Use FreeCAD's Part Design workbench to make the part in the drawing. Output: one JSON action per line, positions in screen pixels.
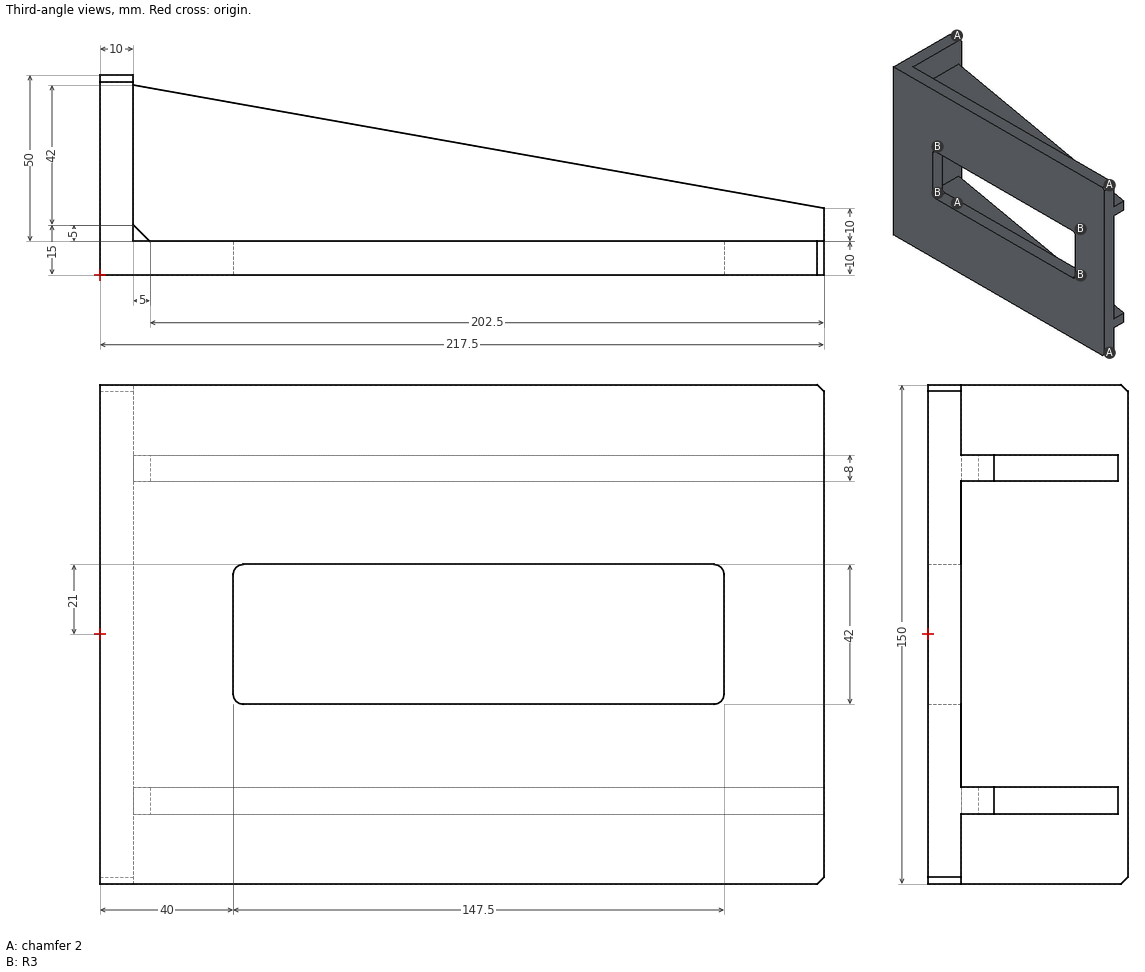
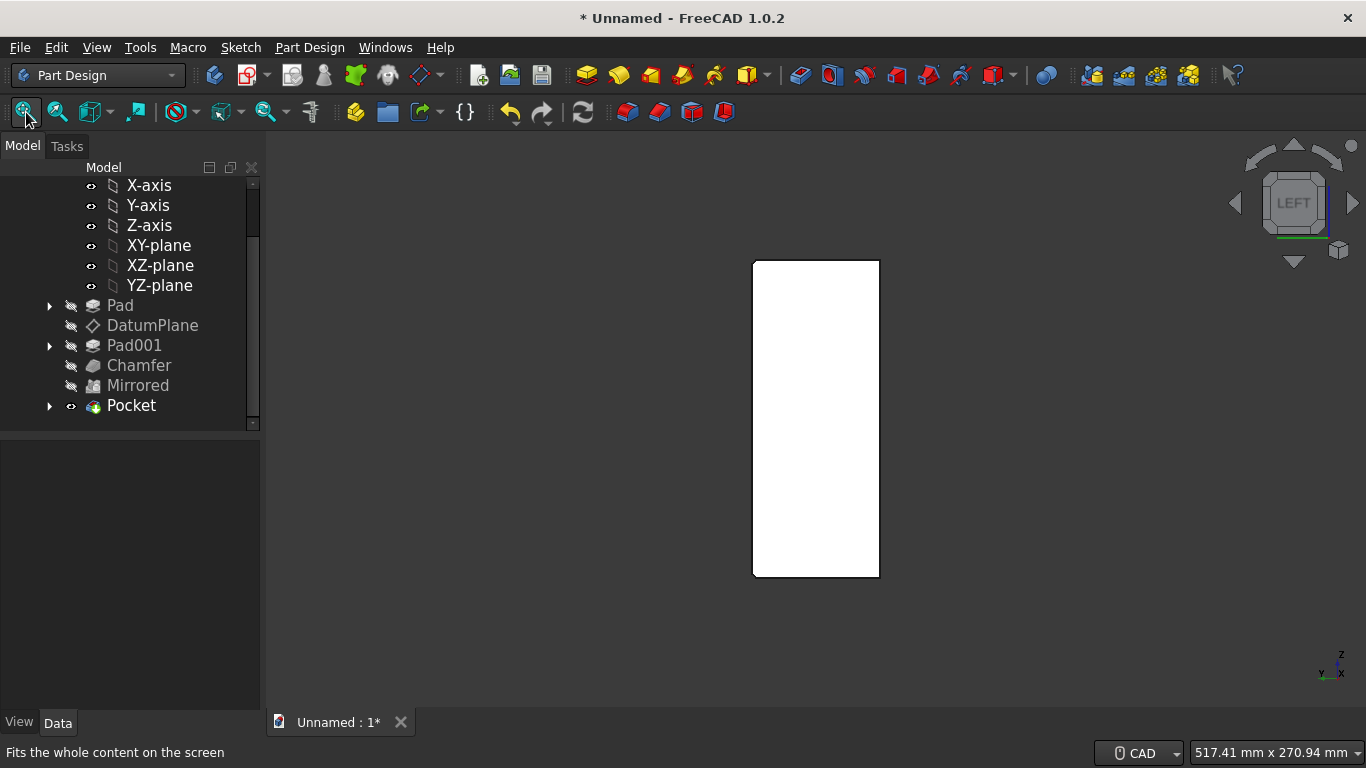
{"action": "scroll", "coordinate": [869, 463], "scroll_direction": "up", "scroll_amount": 4}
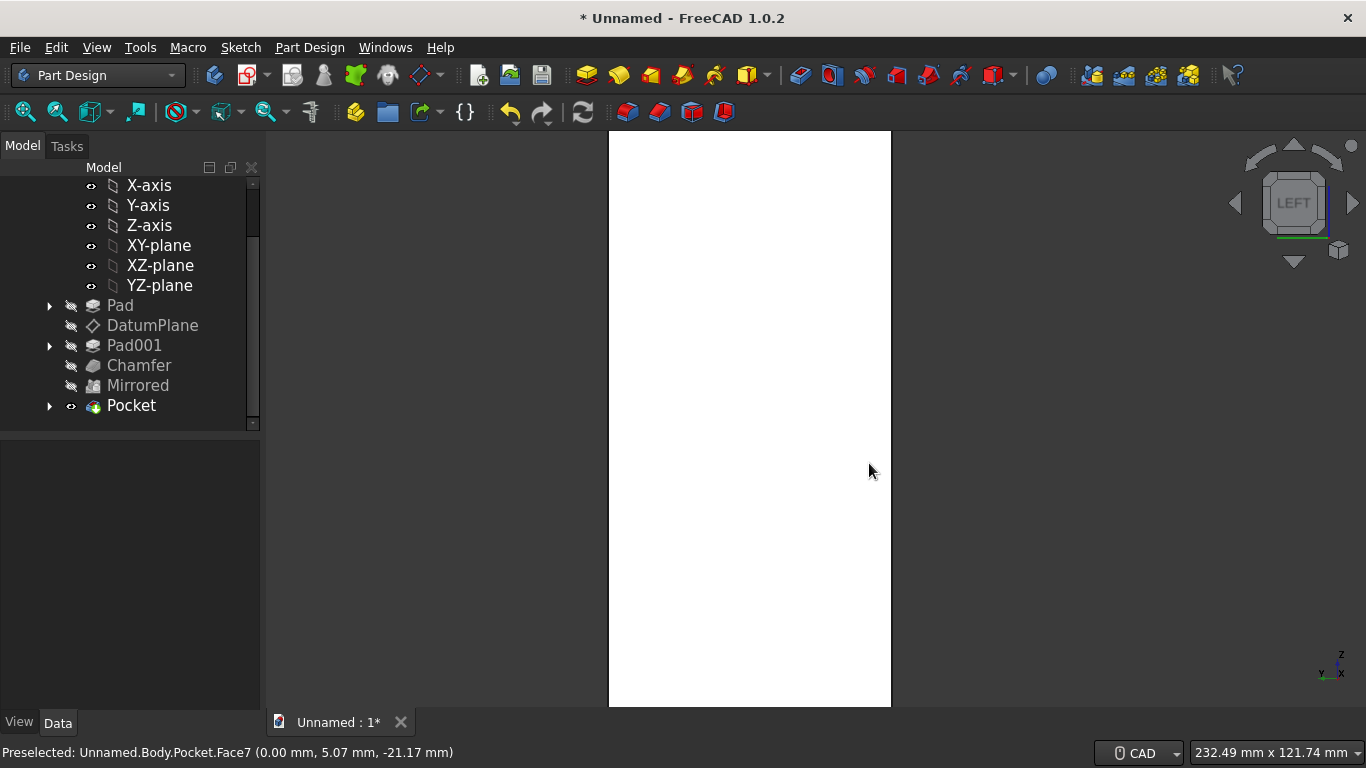
{"action": "left_click", "coordinate": [26, 112]}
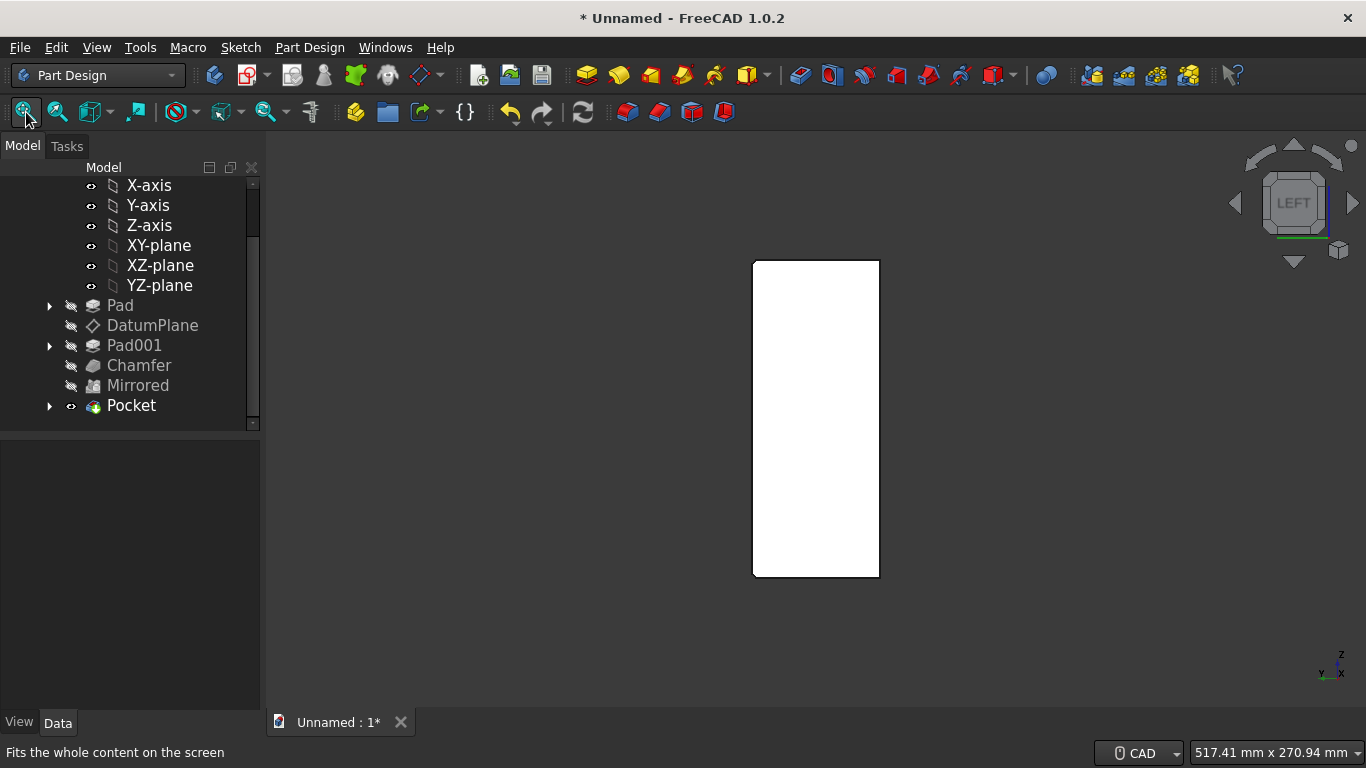
{"action": "key", "text": "v 3"}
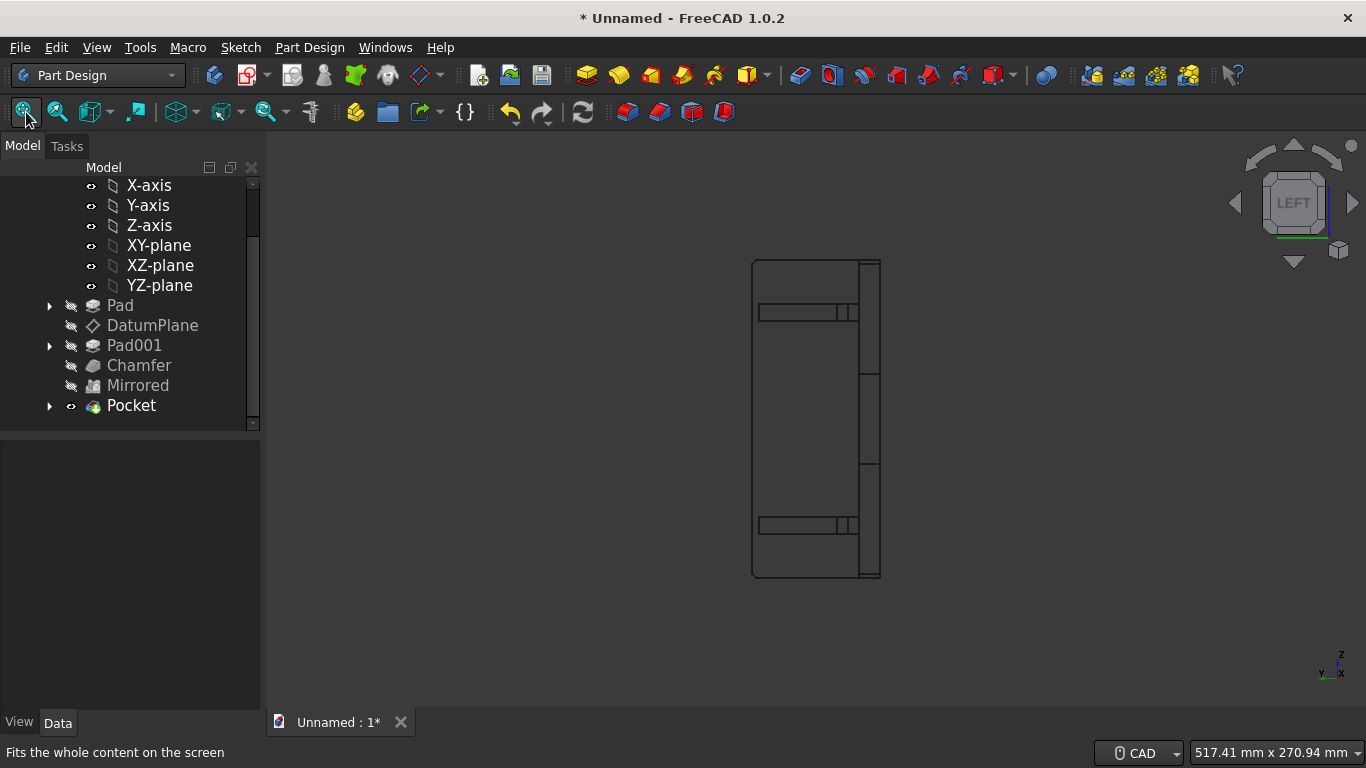
{"action": "key", "text": "0"}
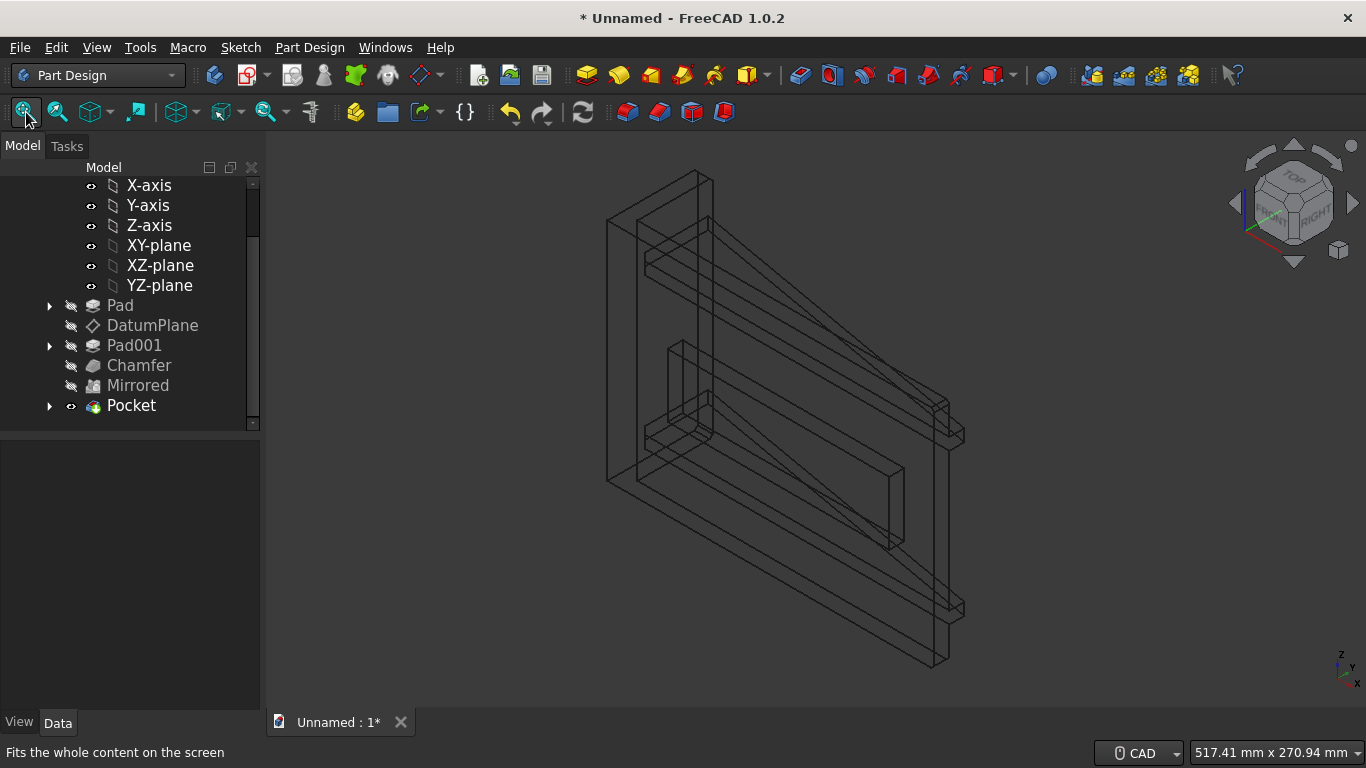
{"action": "left_click", "coordinate": [897, 544]}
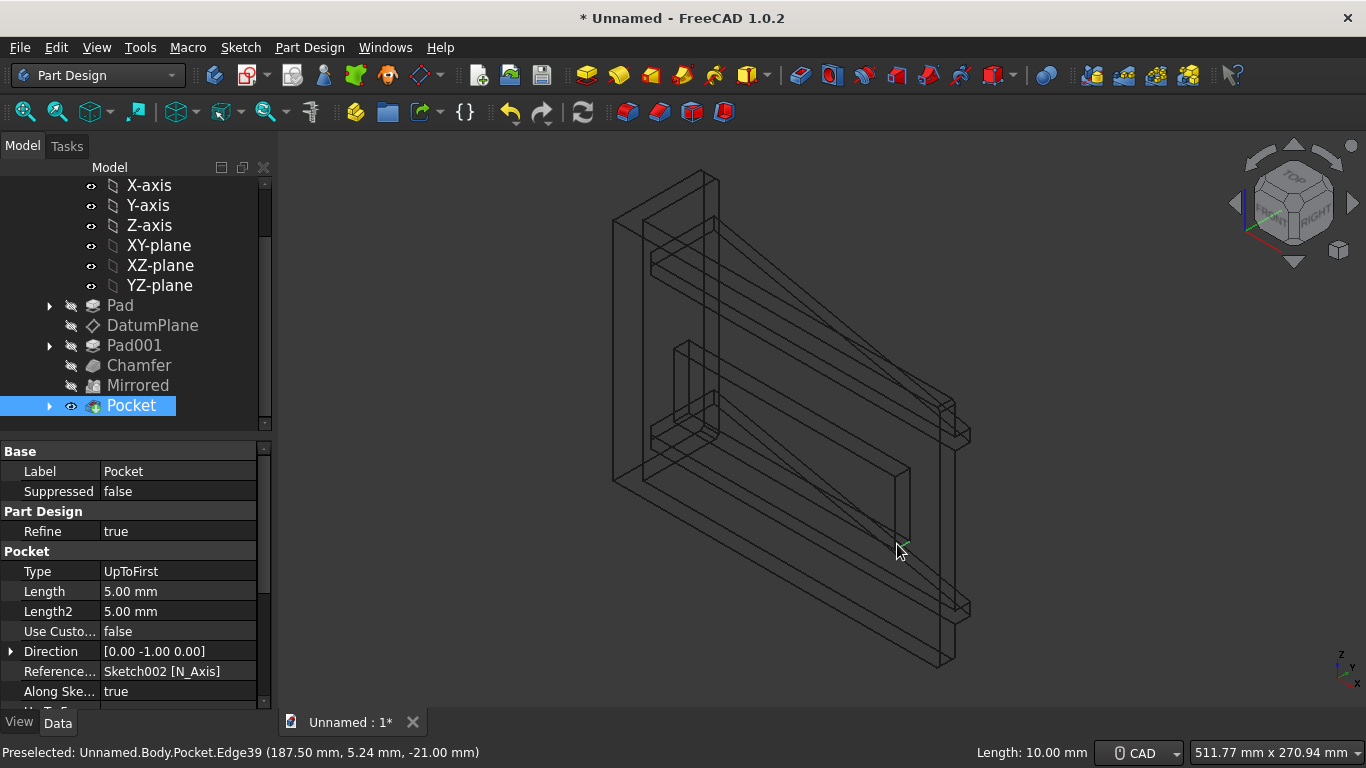
{"action": "left_click", "coordinate": [903, 472], "text": "ctrl"}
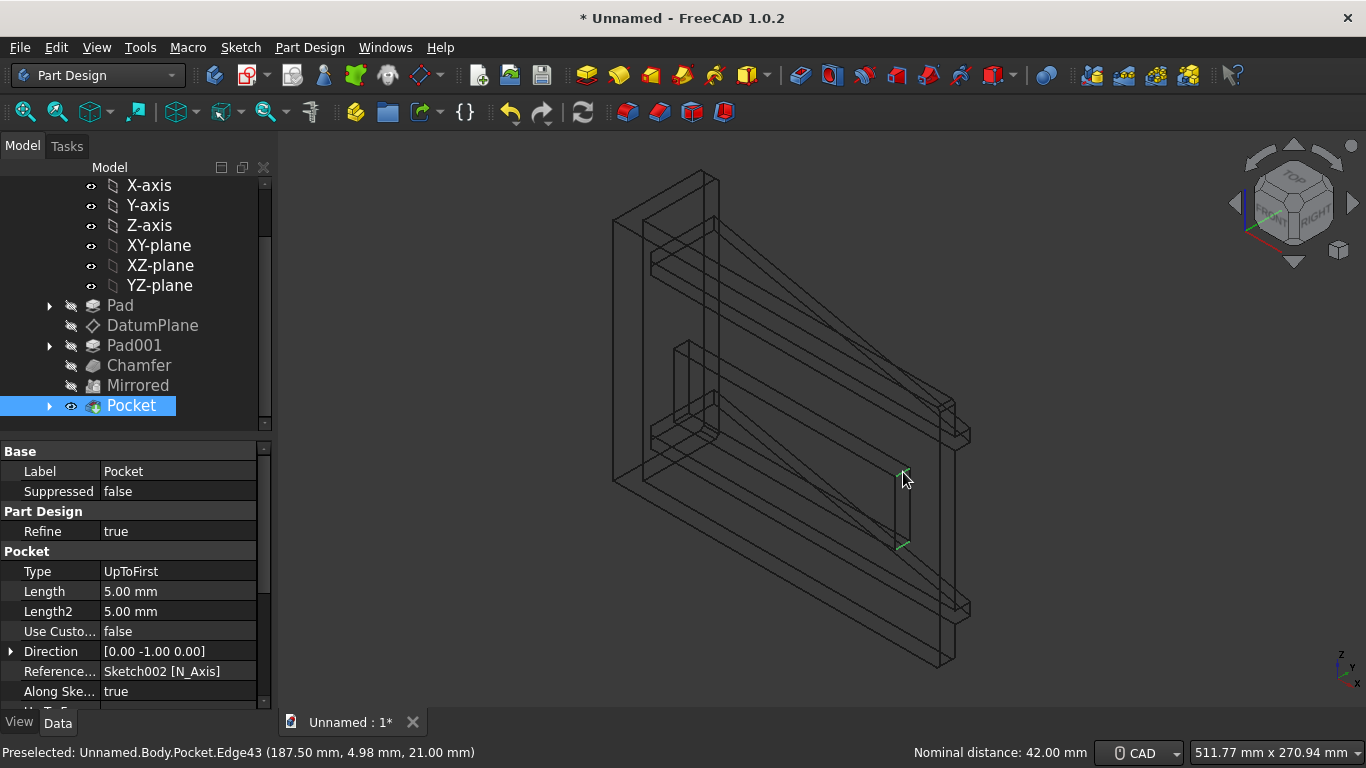
{"action": "left_click", "coordinate": [681, 344], "text": "ctrl"}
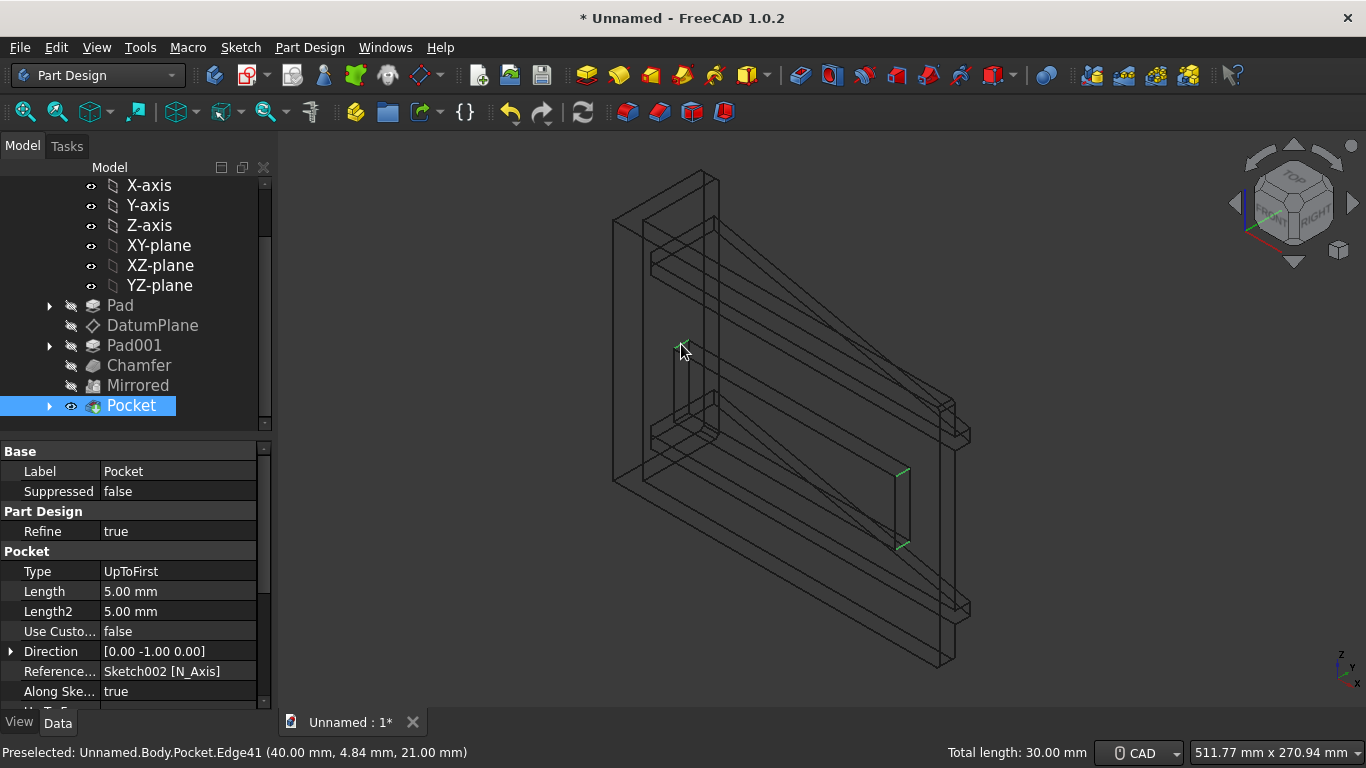
{"action": "left_click", "coordinate": [681, 416], "text": "ctrl"}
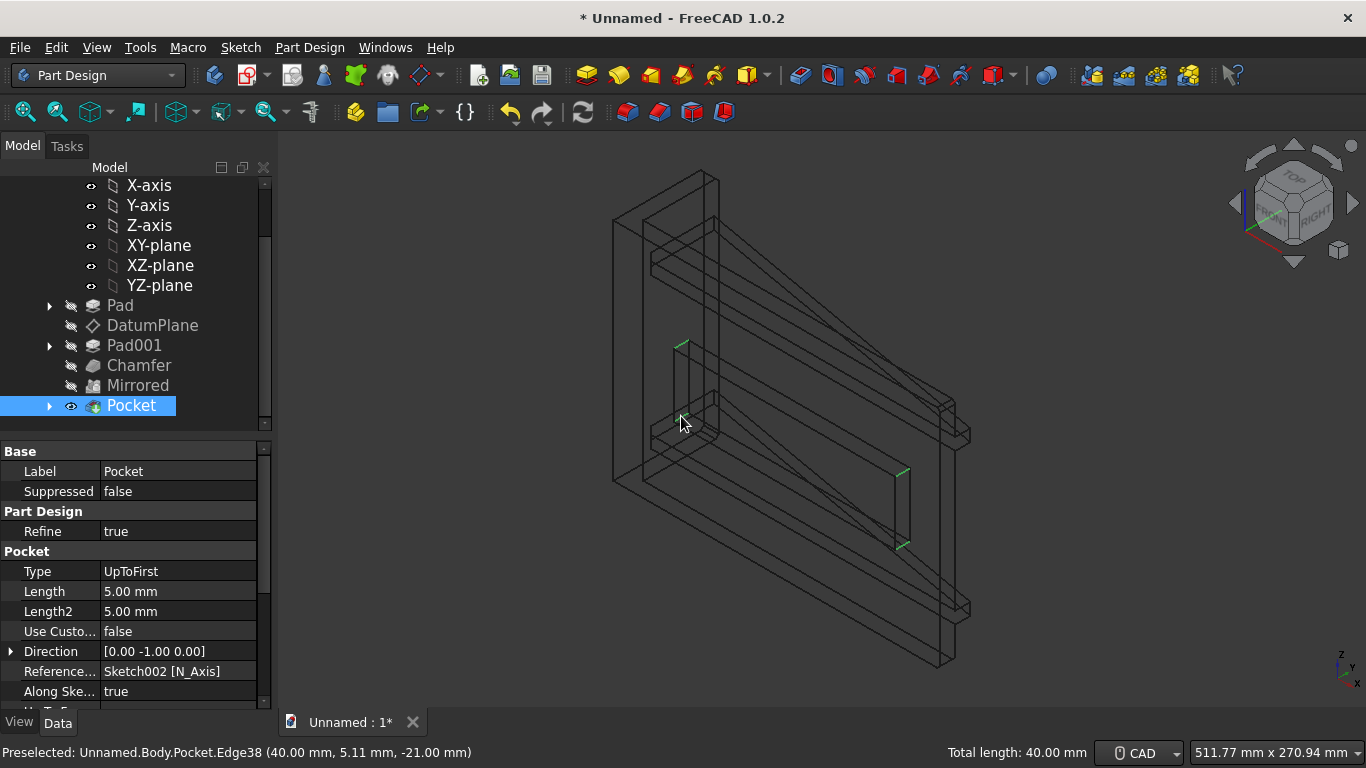
{"action": "key", "text": "v 1"}